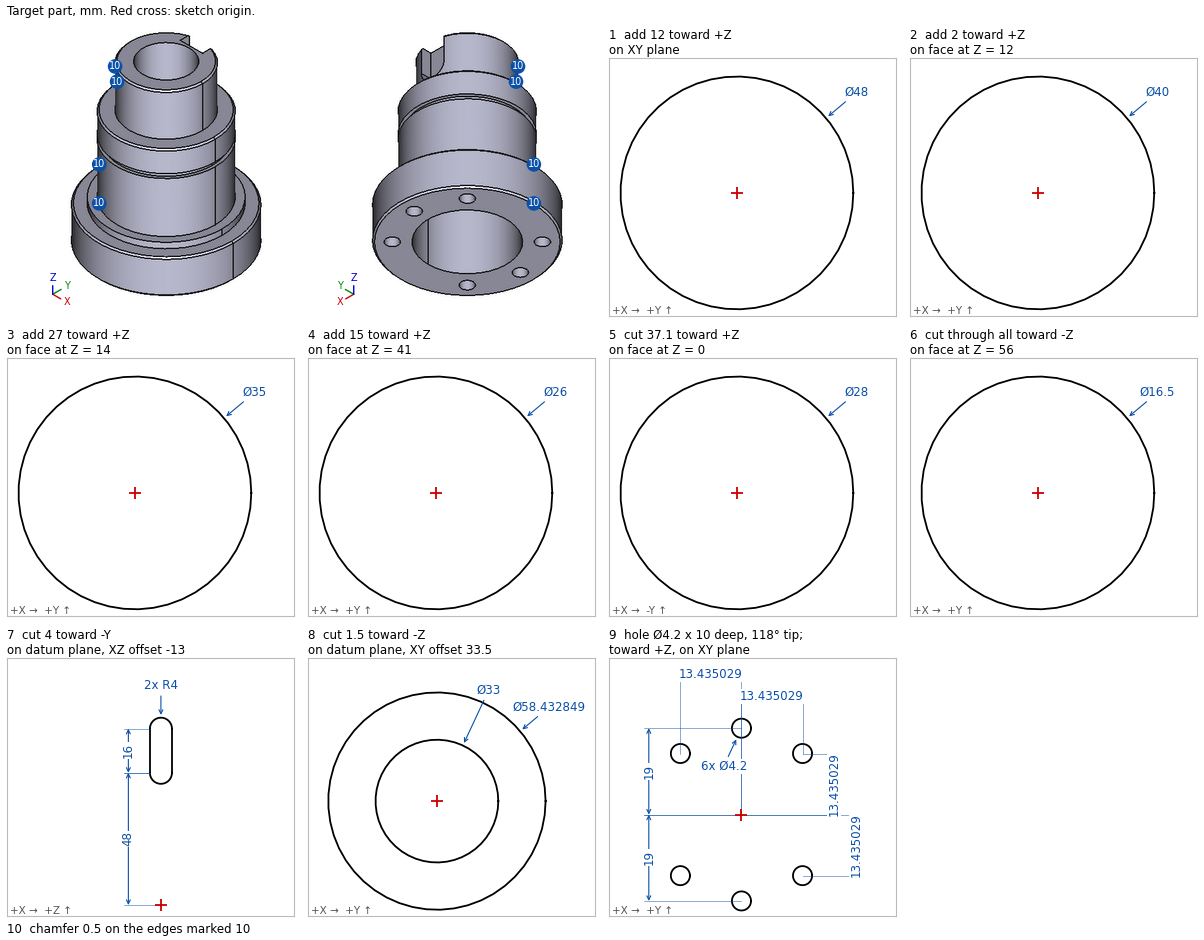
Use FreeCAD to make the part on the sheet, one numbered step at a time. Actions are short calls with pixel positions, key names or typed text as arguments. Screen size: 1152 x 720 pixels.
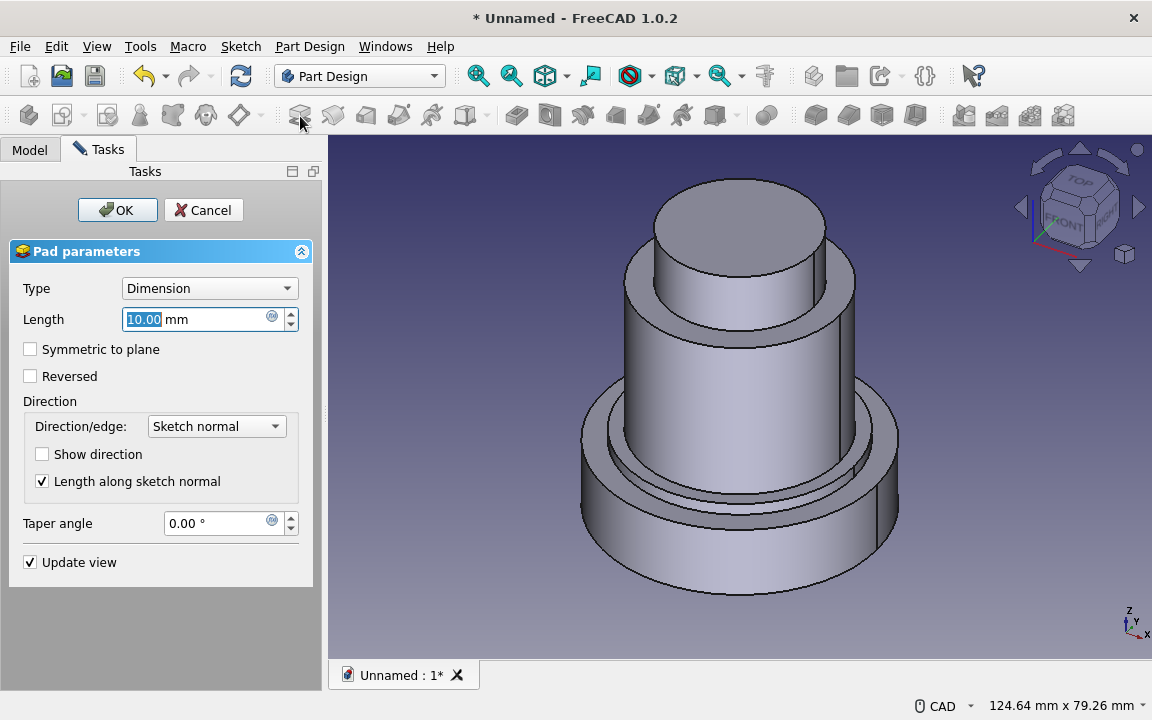
text(15)
key(Tab)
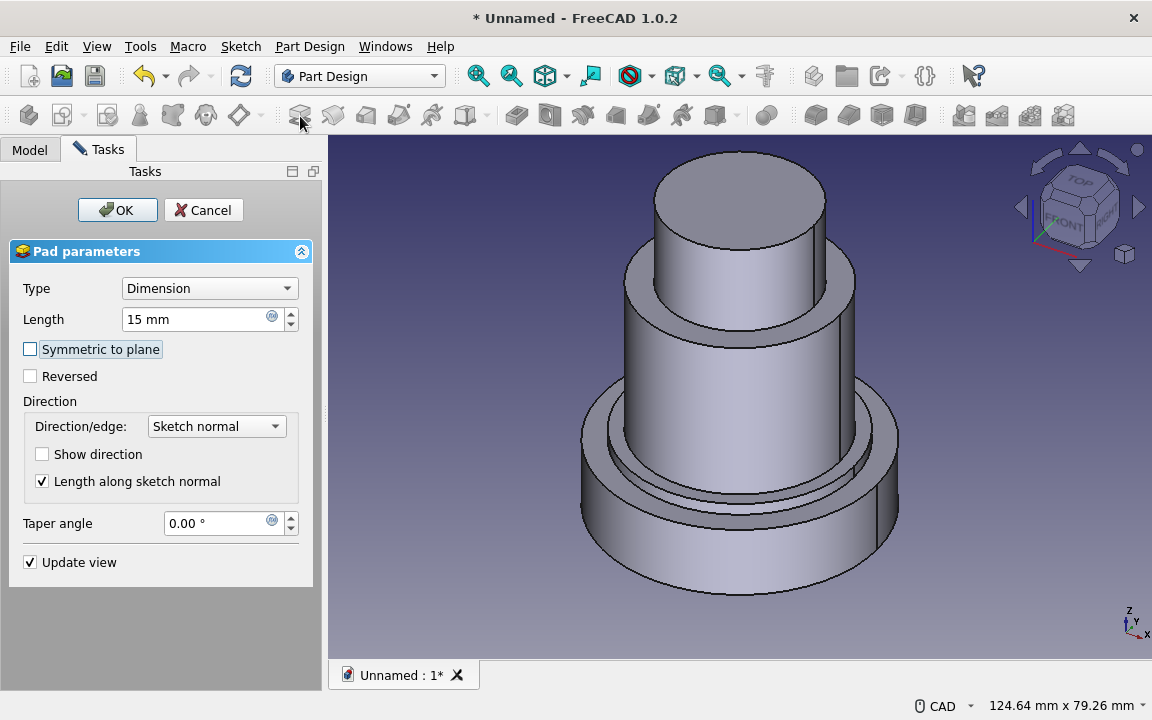
click(118, 210)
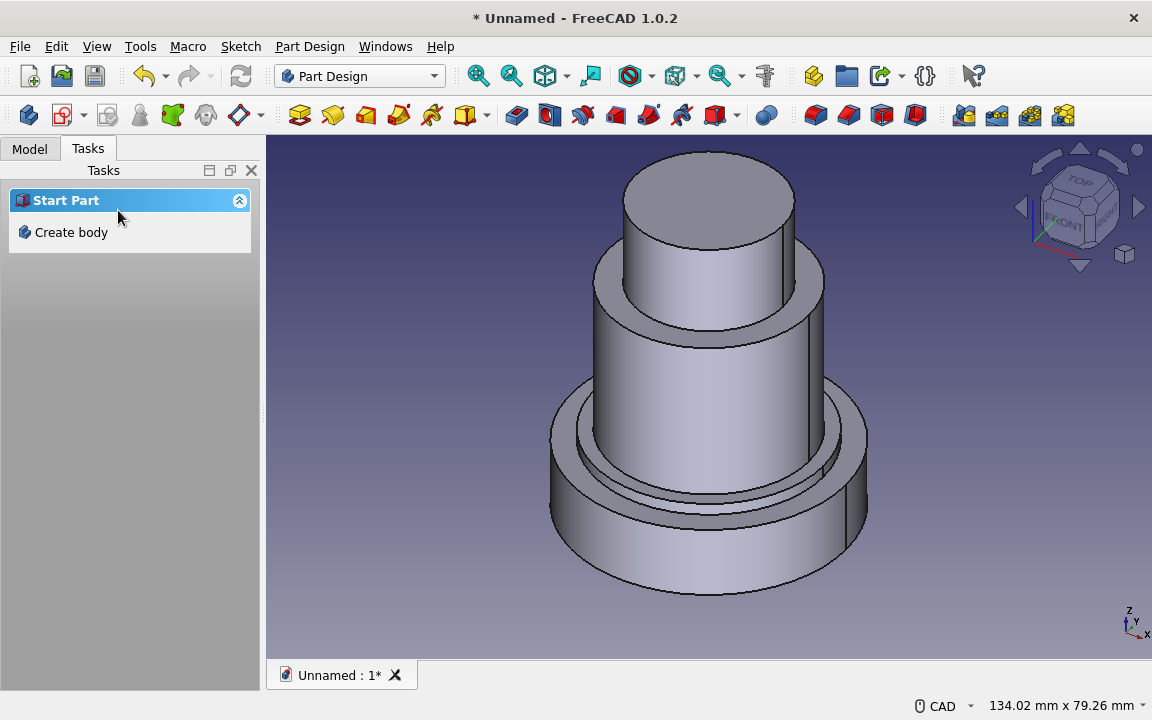
click(479, 76)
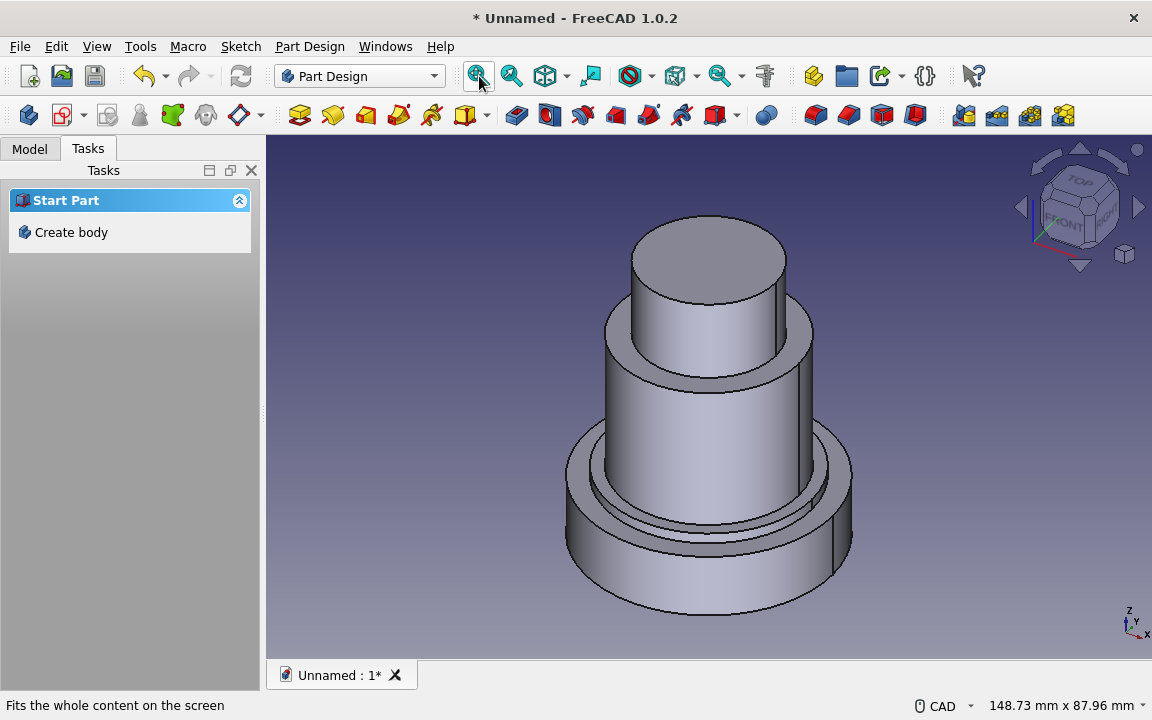
key(5)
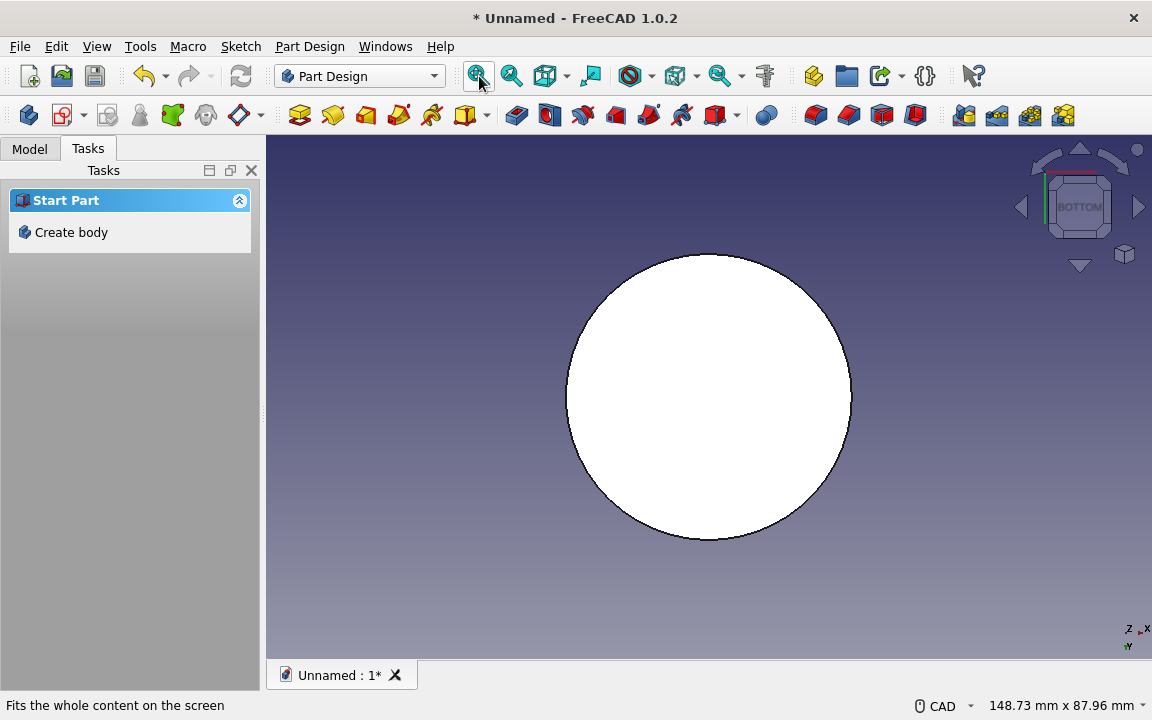
click(709, 396)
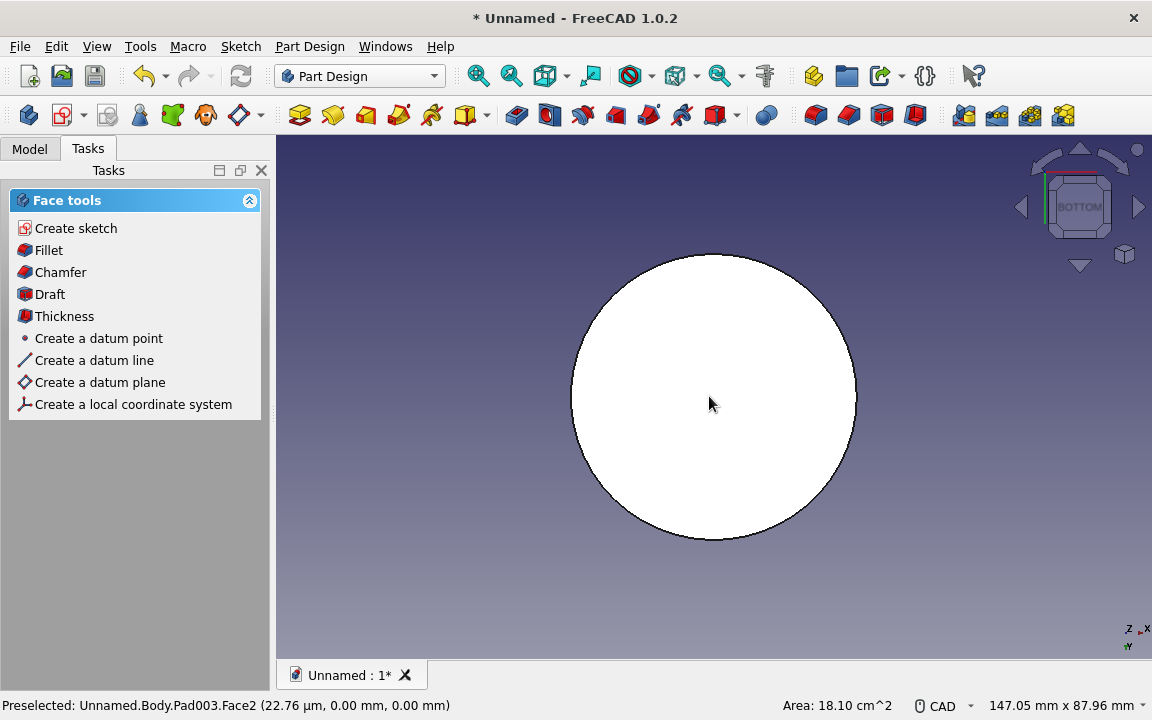
click(62, 116)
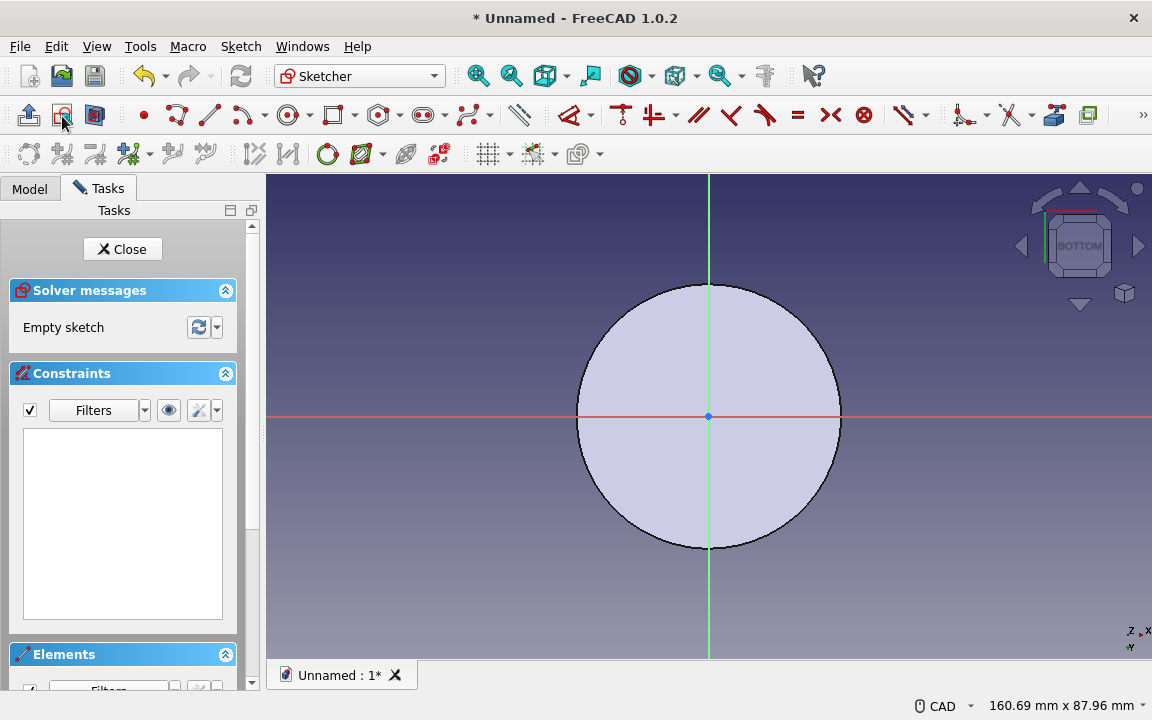
scroll(792, 416, up, 3)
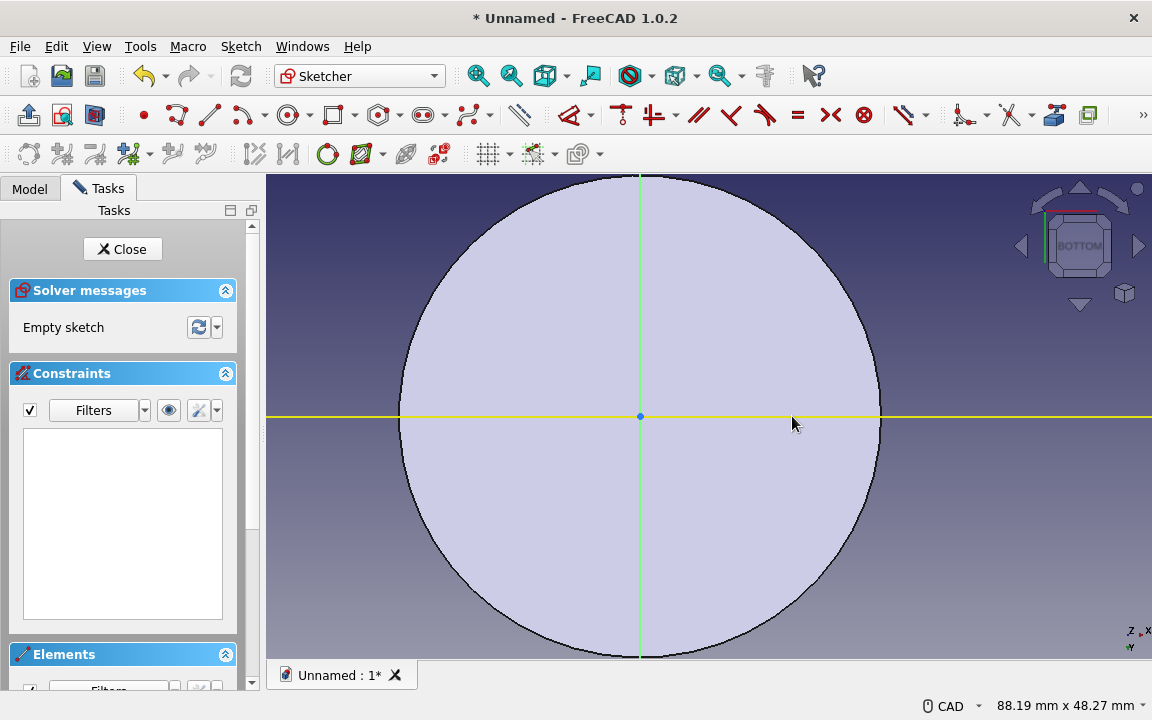
key(g)
key(c)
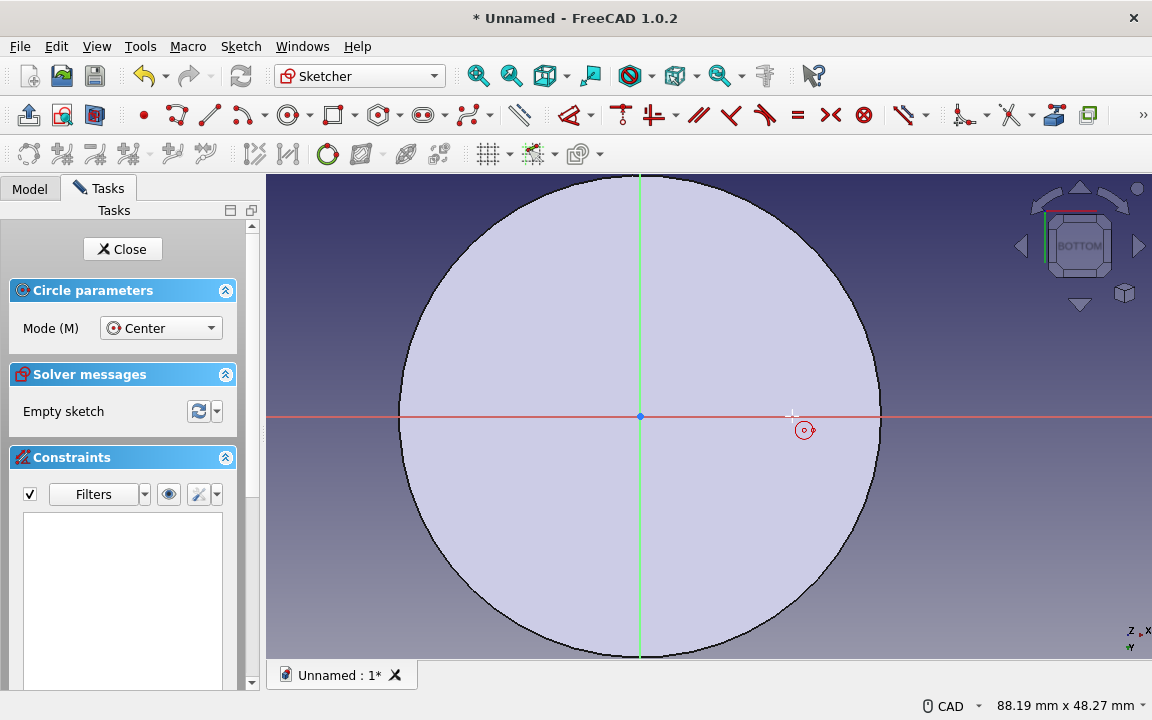
click(640, 416)
click(740, 317)
key(Escape)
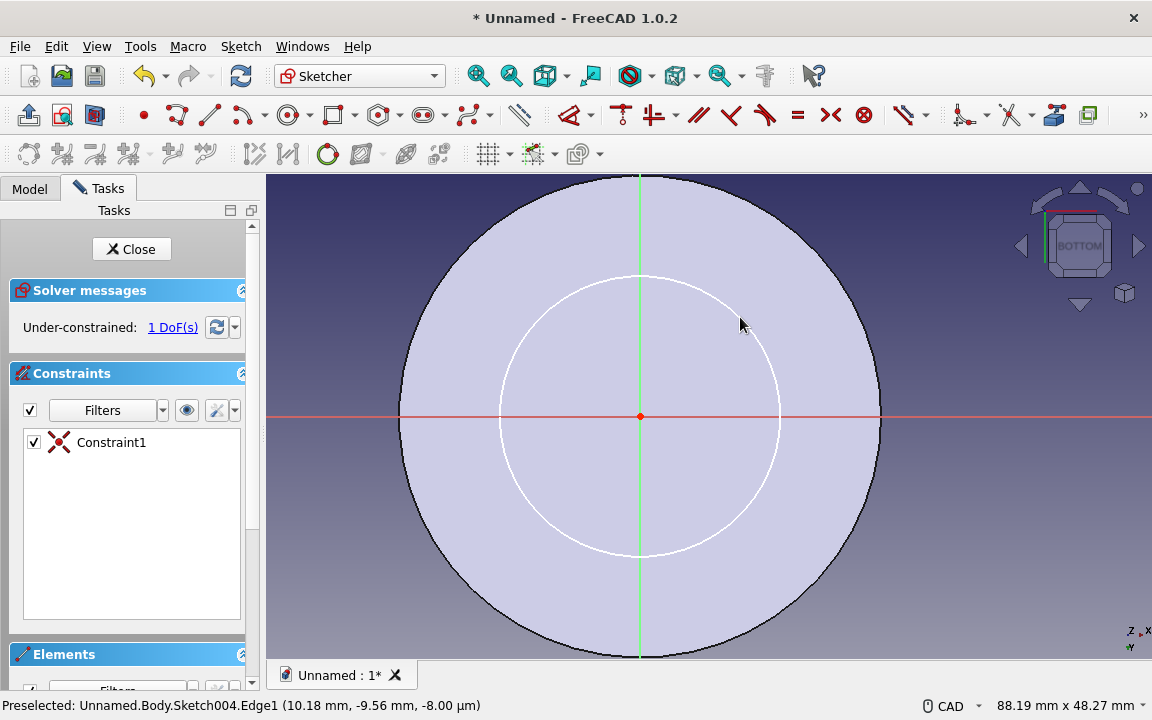
click(739, 317)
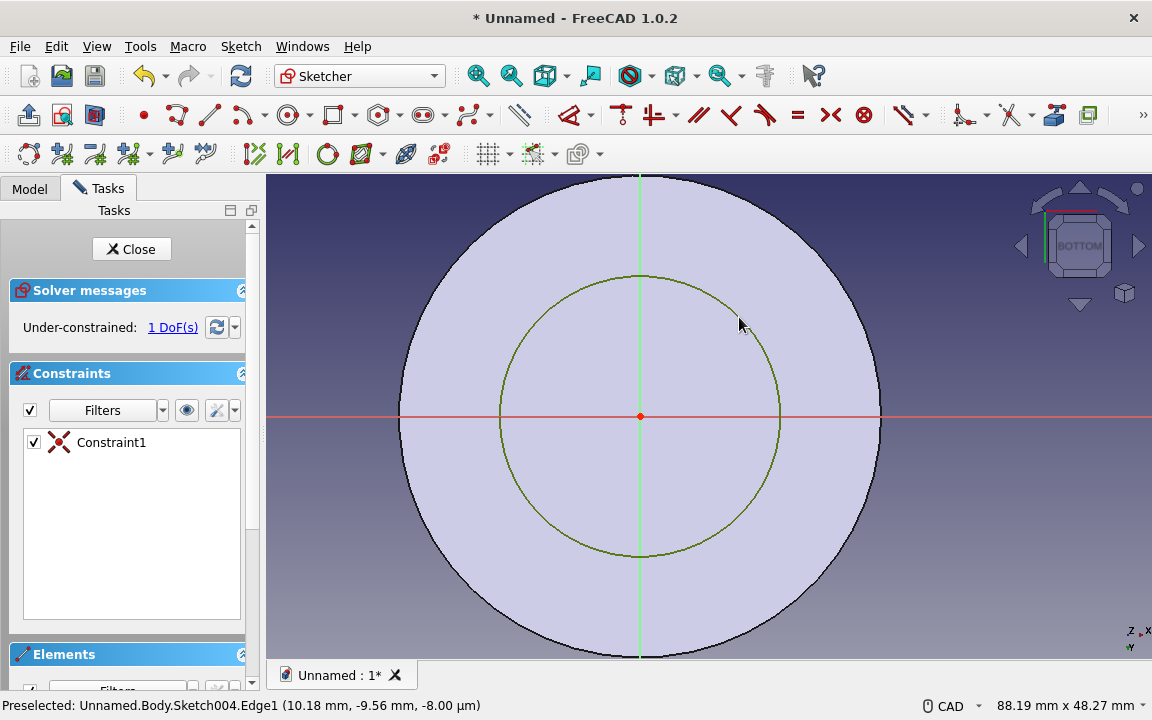
key(k)
key(o)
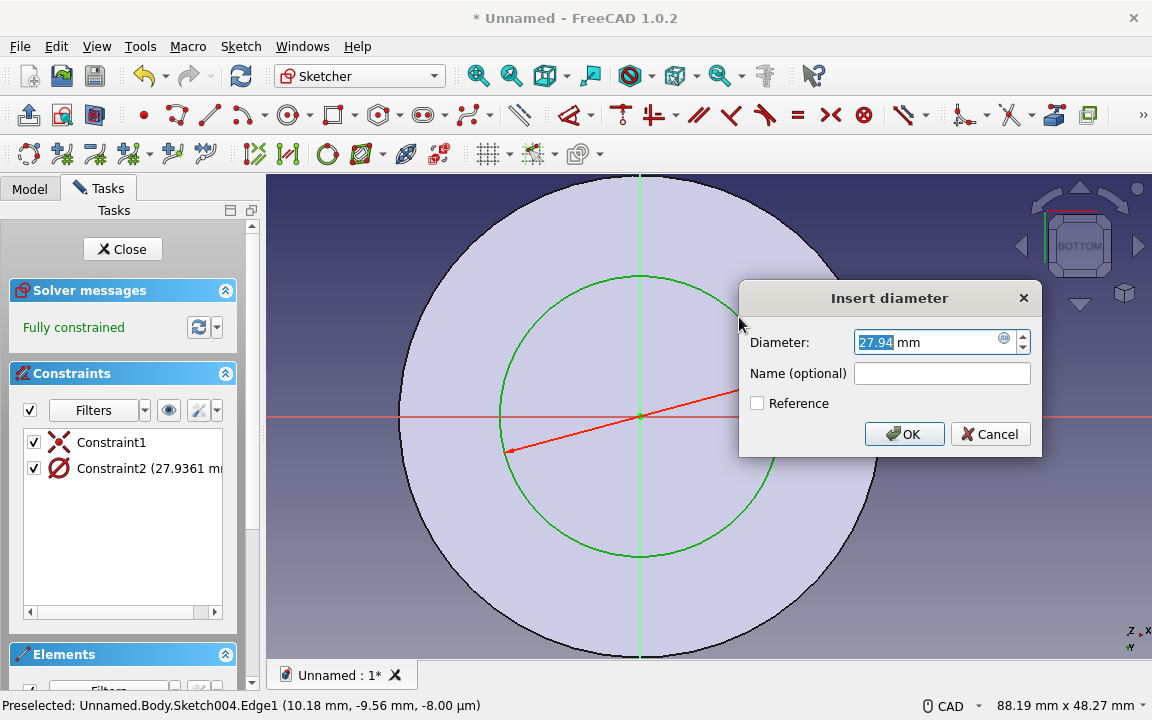
text(28)
key(Return)